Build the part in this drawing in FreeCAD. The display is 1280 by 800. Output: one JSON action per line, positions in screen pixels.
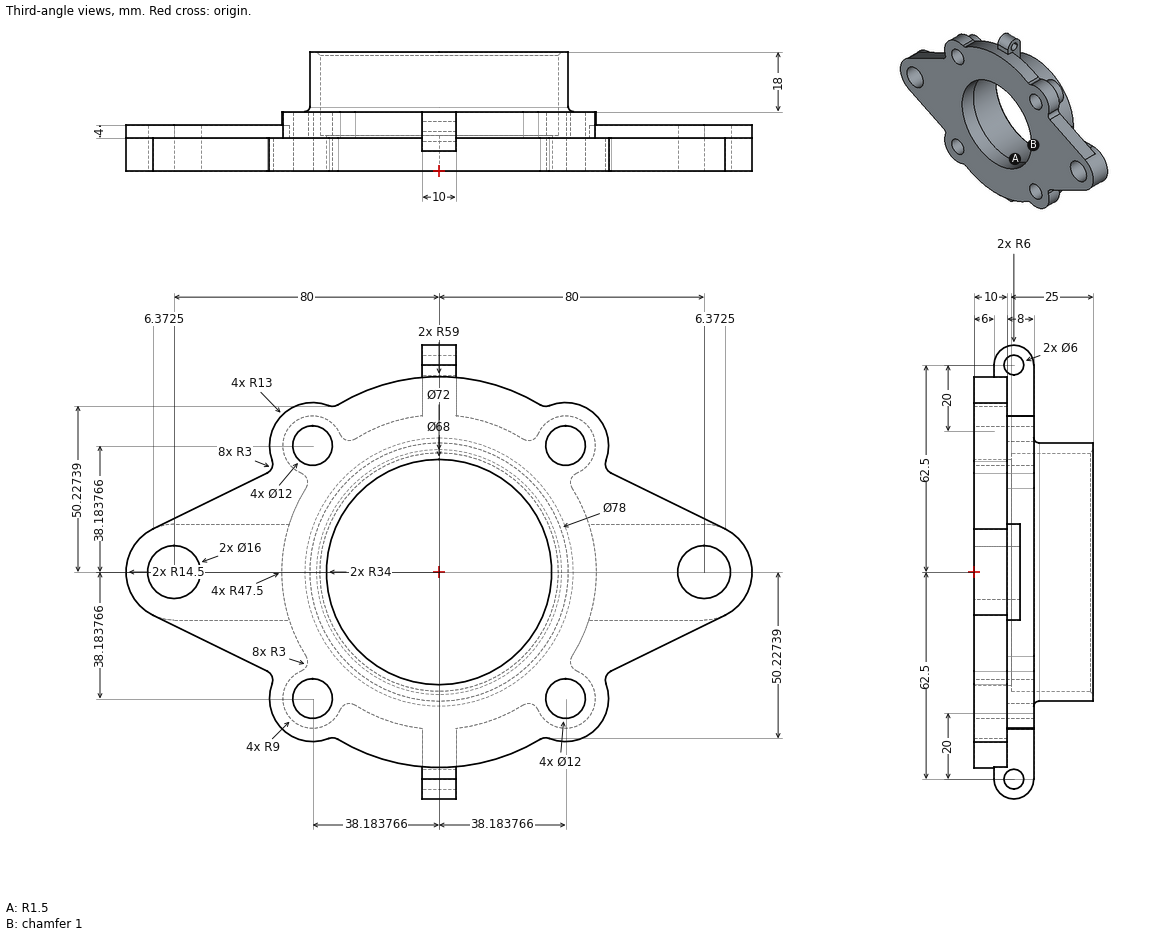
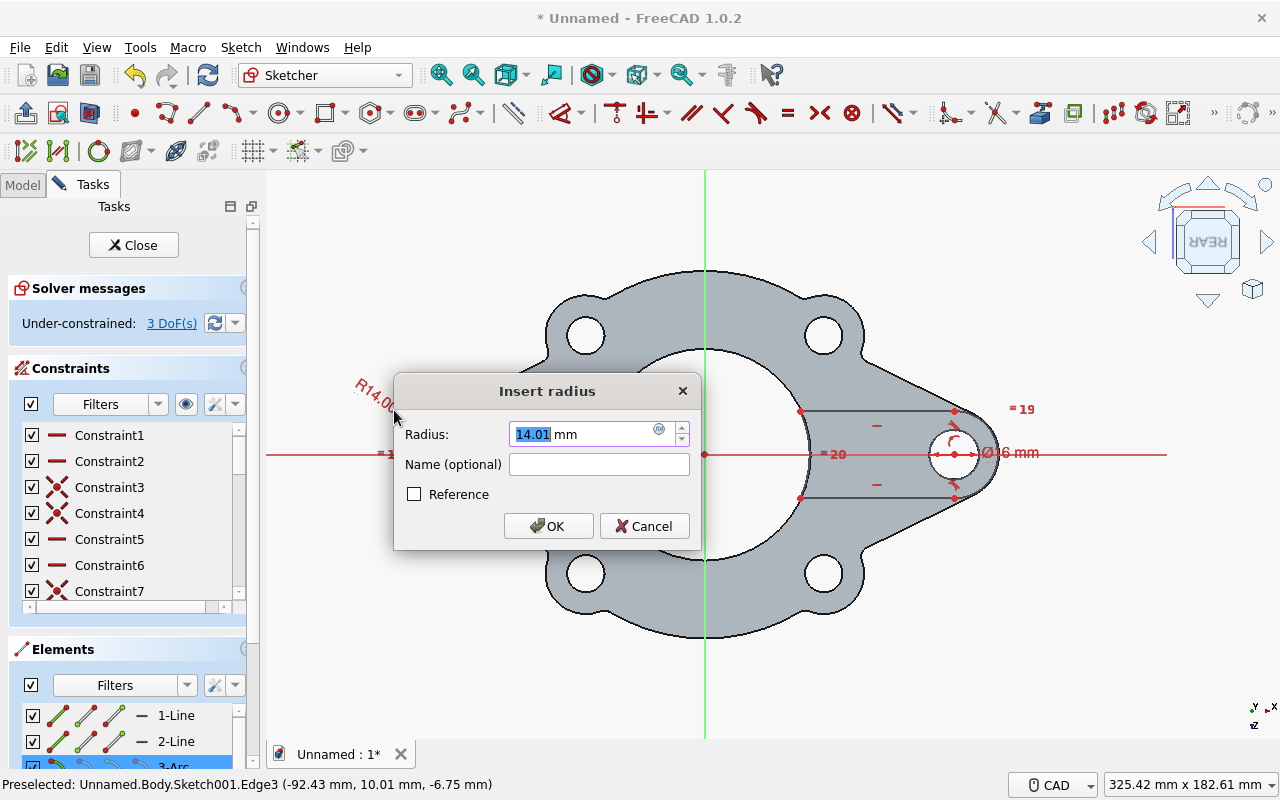
{"action": "type", "text": "14.5"}
{"action": "key", "text": "Return"}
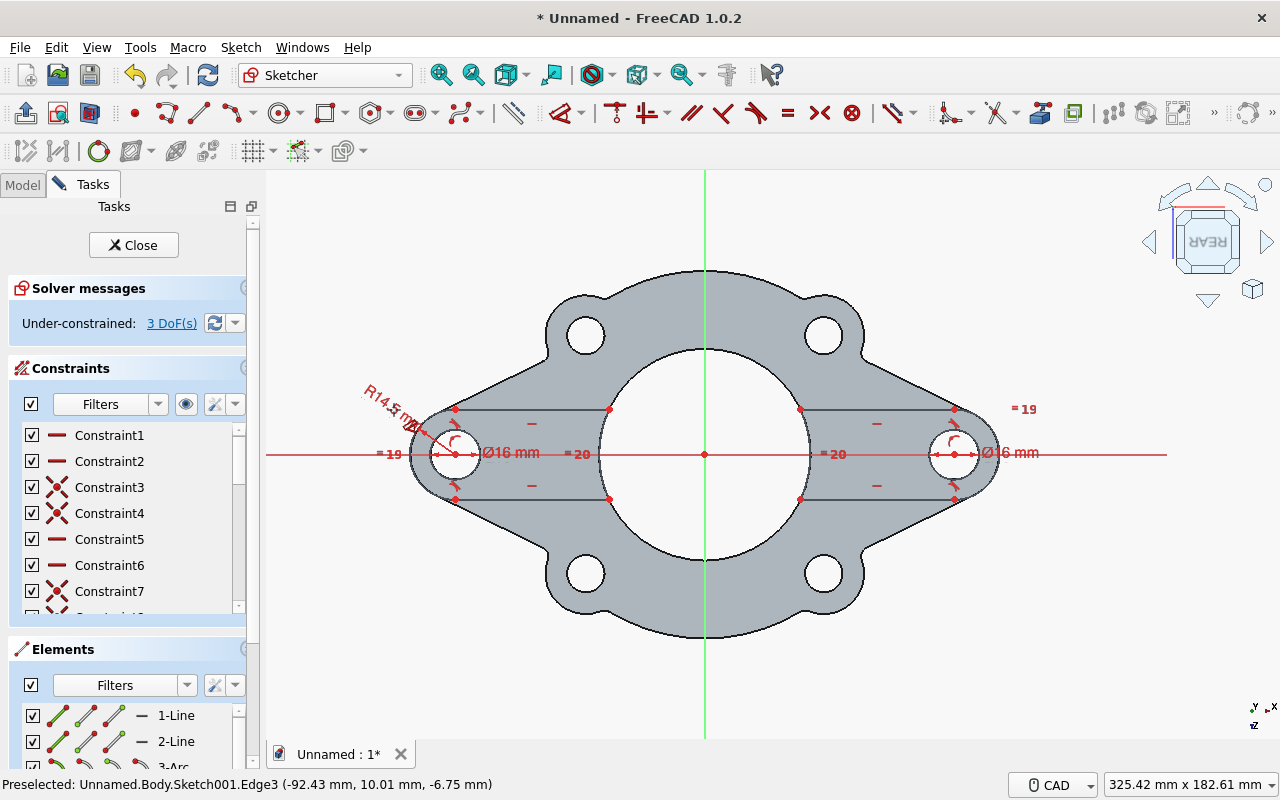
{"action": "left_click", "coordinate": [601, 436]}
{"action": "left_click", "coordinate": [570, 430]}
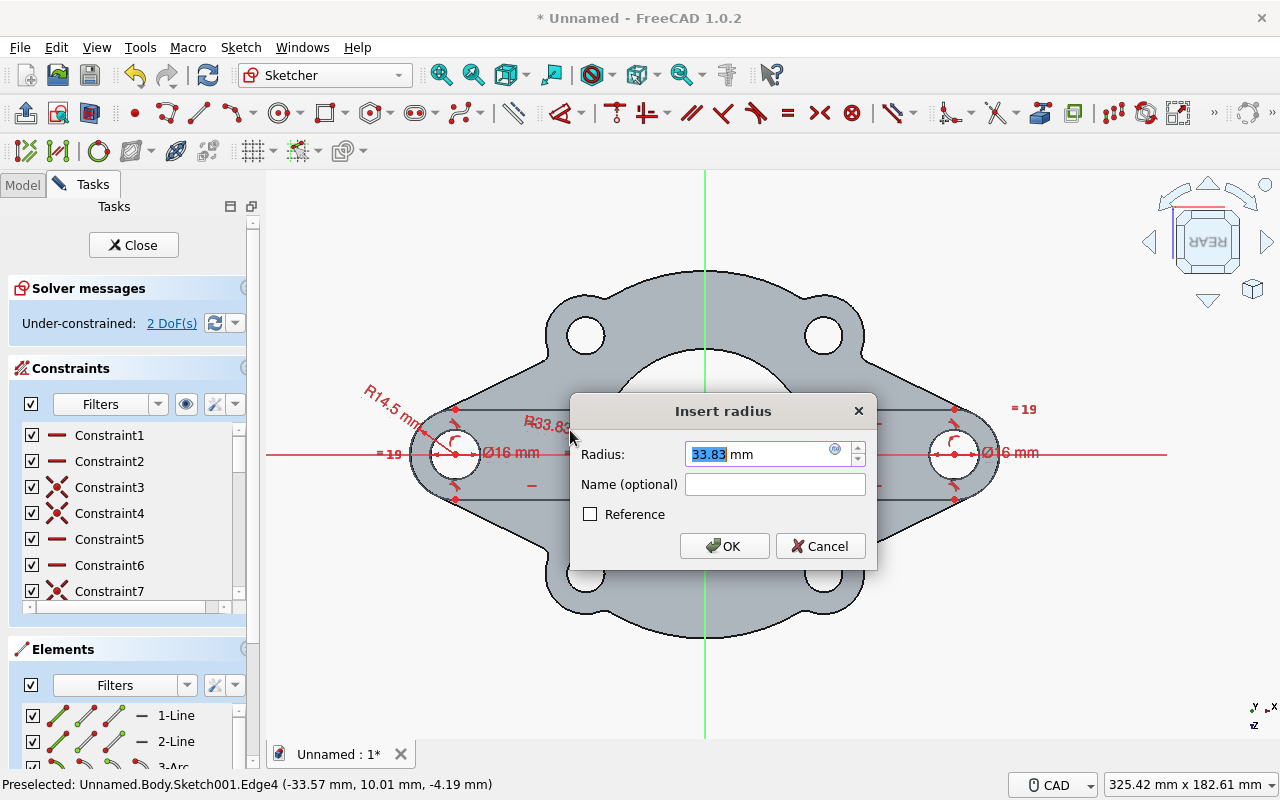
{"action": "type", "text": "34"}
{"action": "key", "text": "Return"}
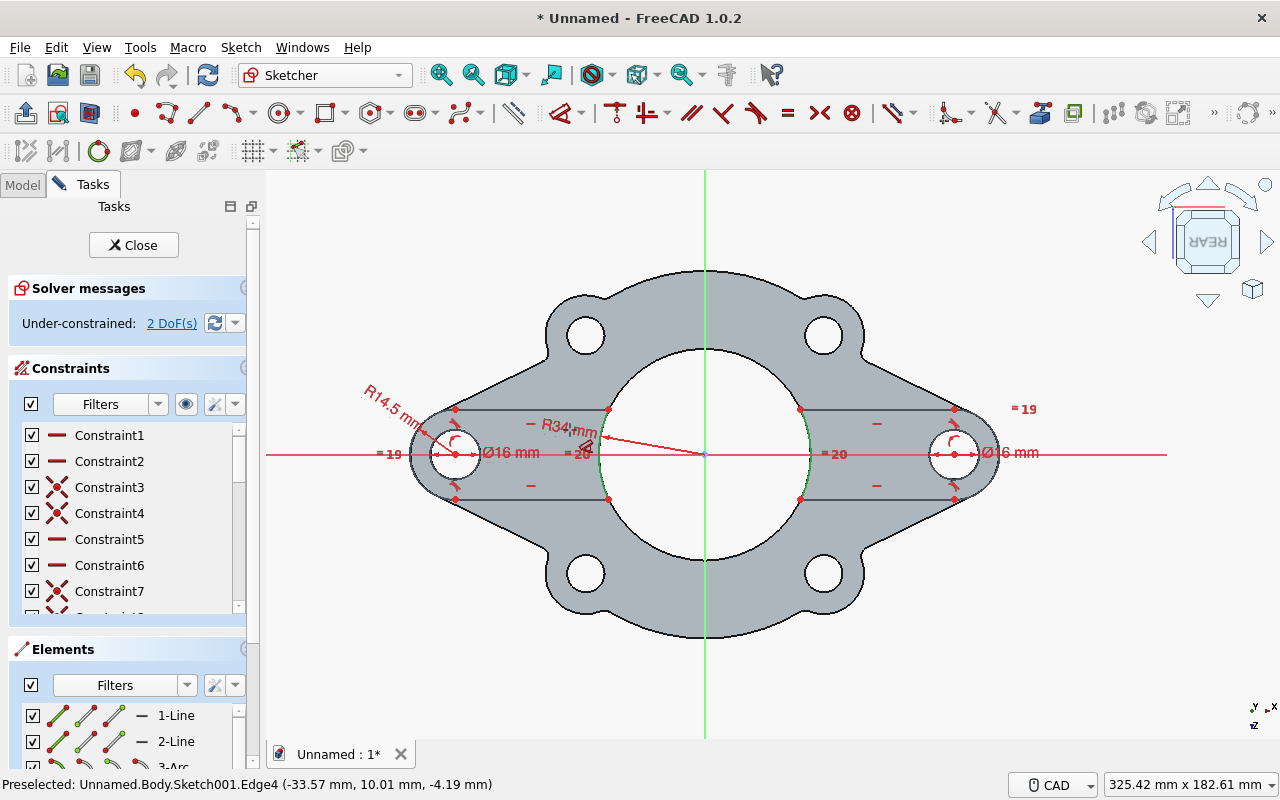
{"action": "left_click", "coordinate": [455, 455]}
{"action": "left_click", "coordinate": [637, 489]}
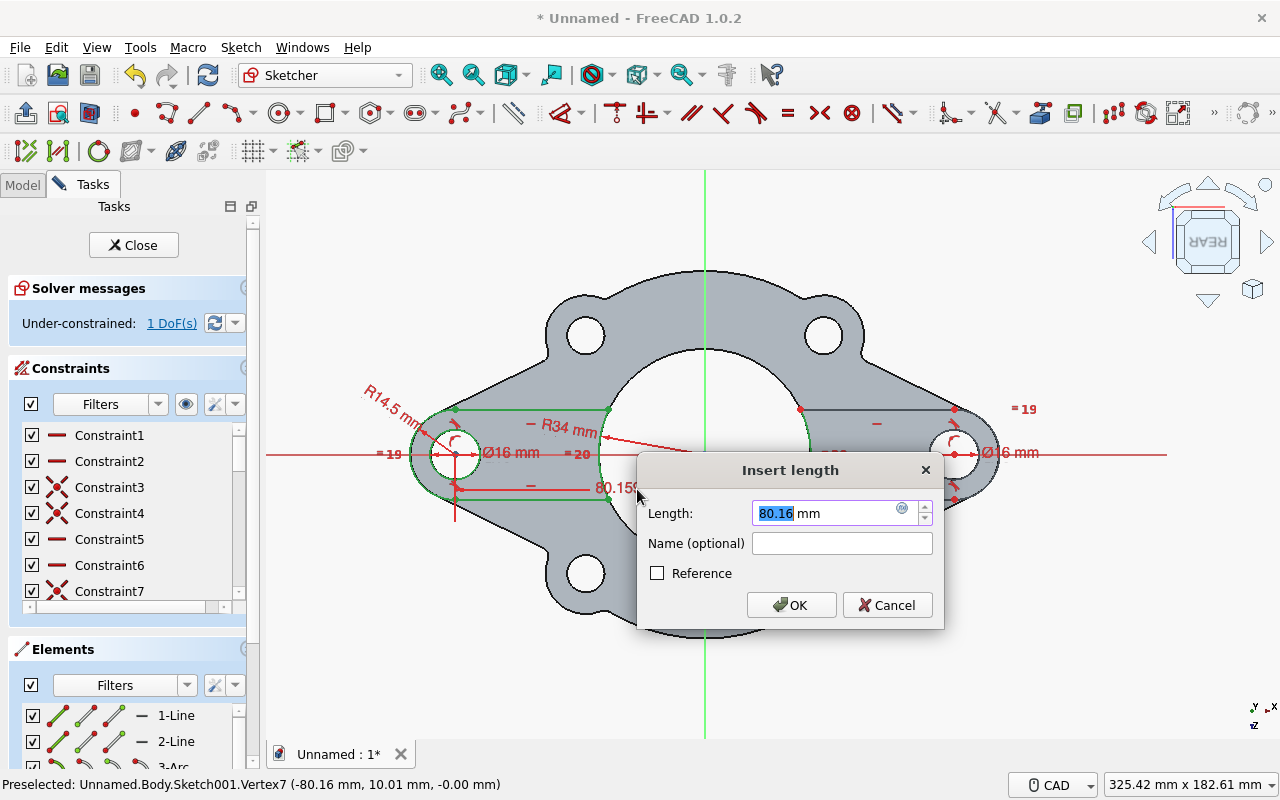
{"action": "type", "text": "80"}
{"action": "key", "text": "Return"}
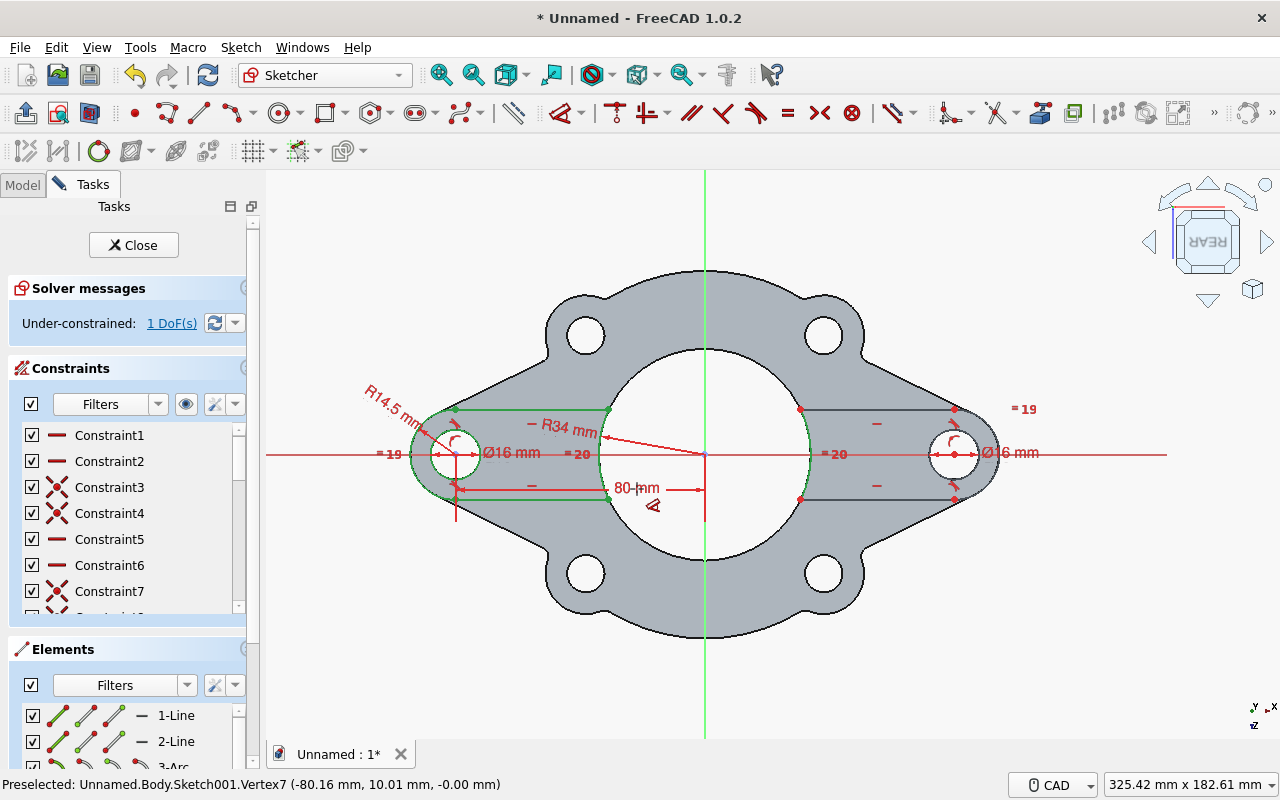
{"action": "left_click", "coordinate": [954, 455]}
{"action": "left_click", "coordinate": [772, 489]}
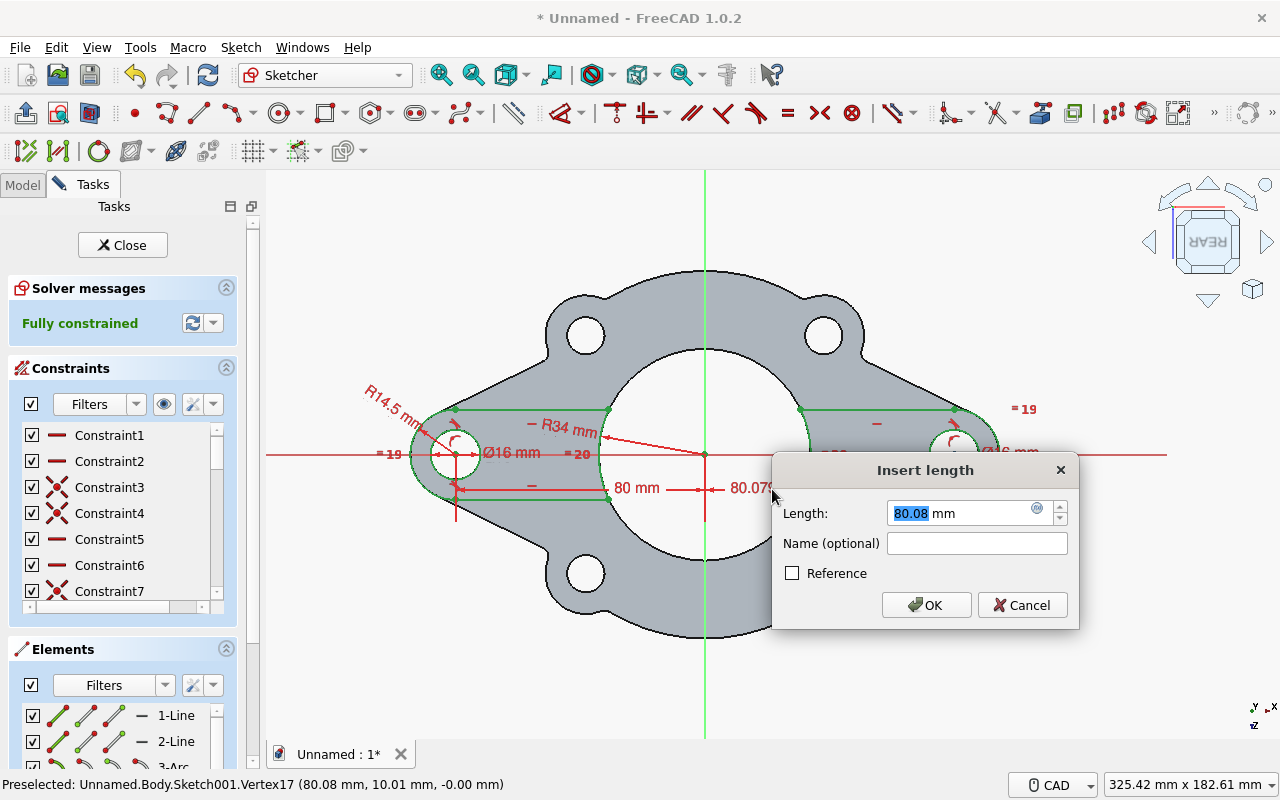
{"action": "type", "text": "80"}
{"action": "key", "text": "Return"}
{"action": "key", "text": "Escape"}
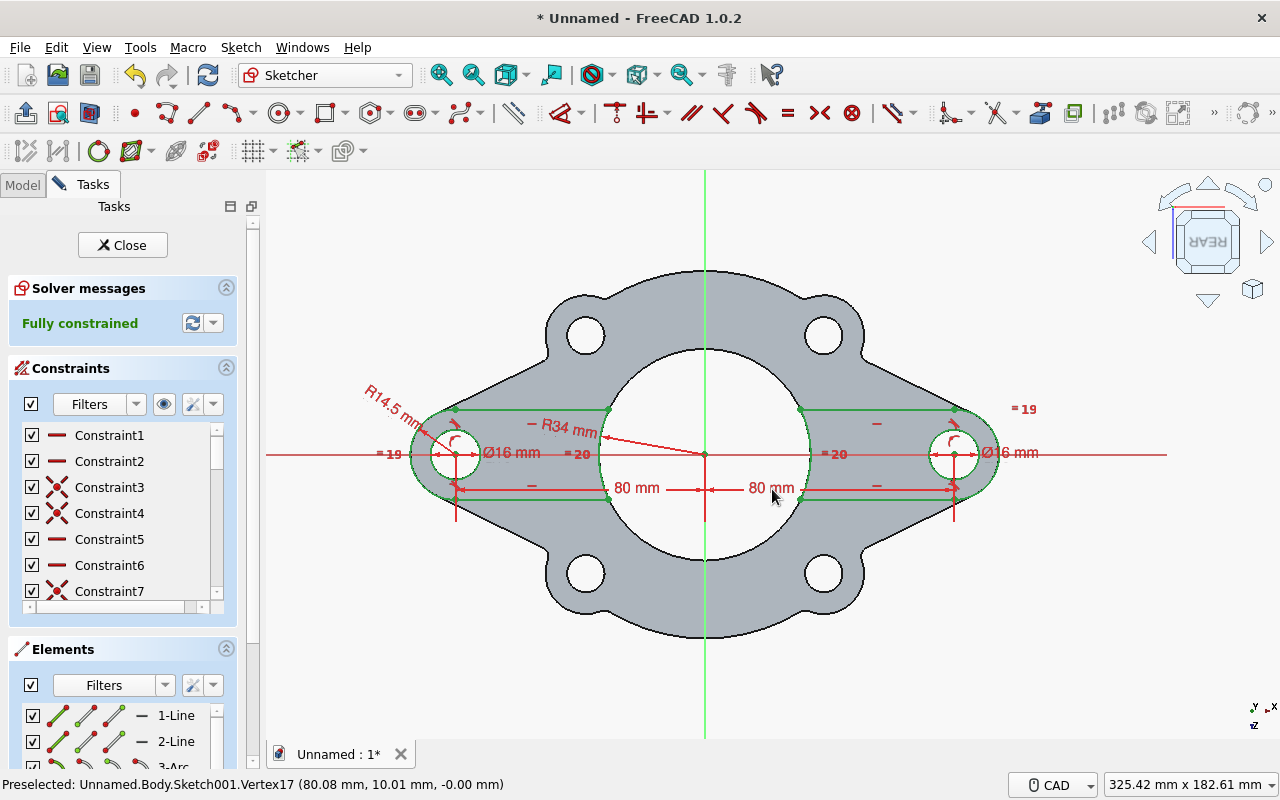
{"action": "left_click", "coordinate": [123, 245]}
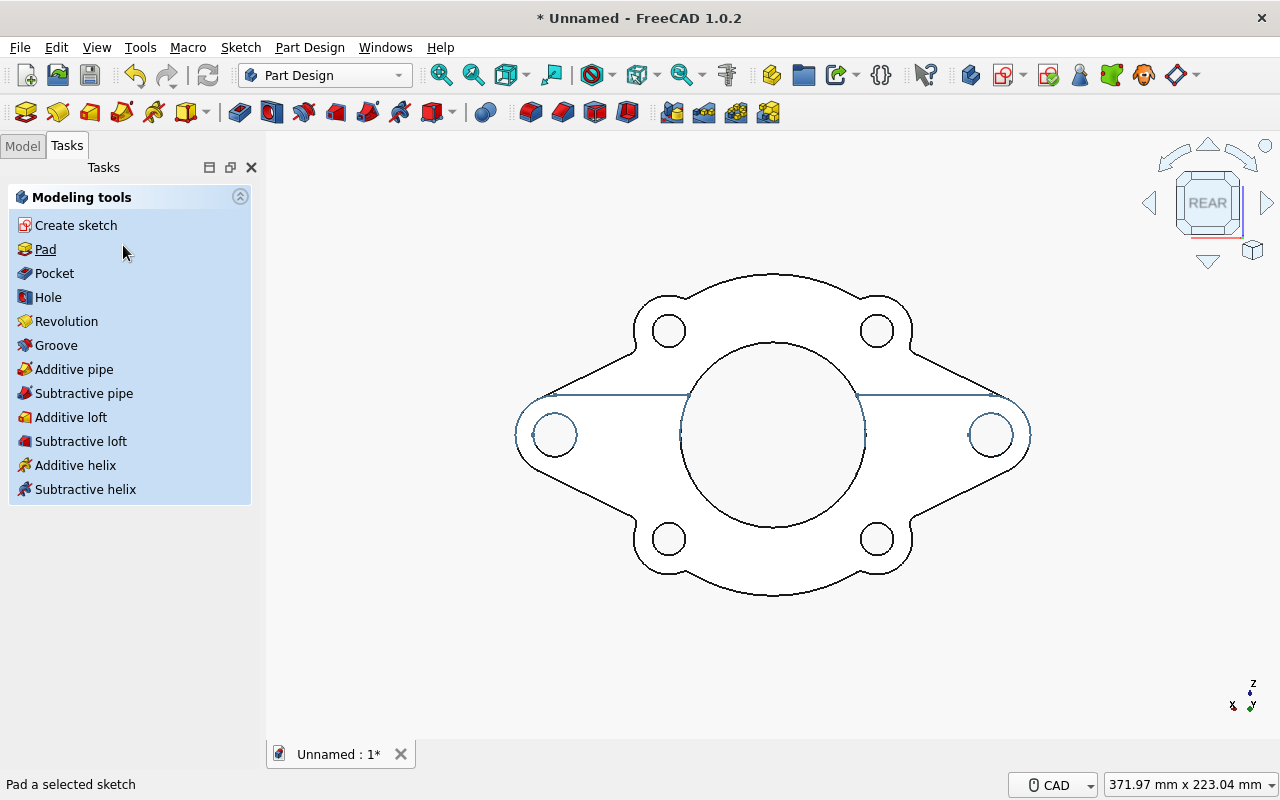
{"action": "left_click", "coordinate": [26, 112]}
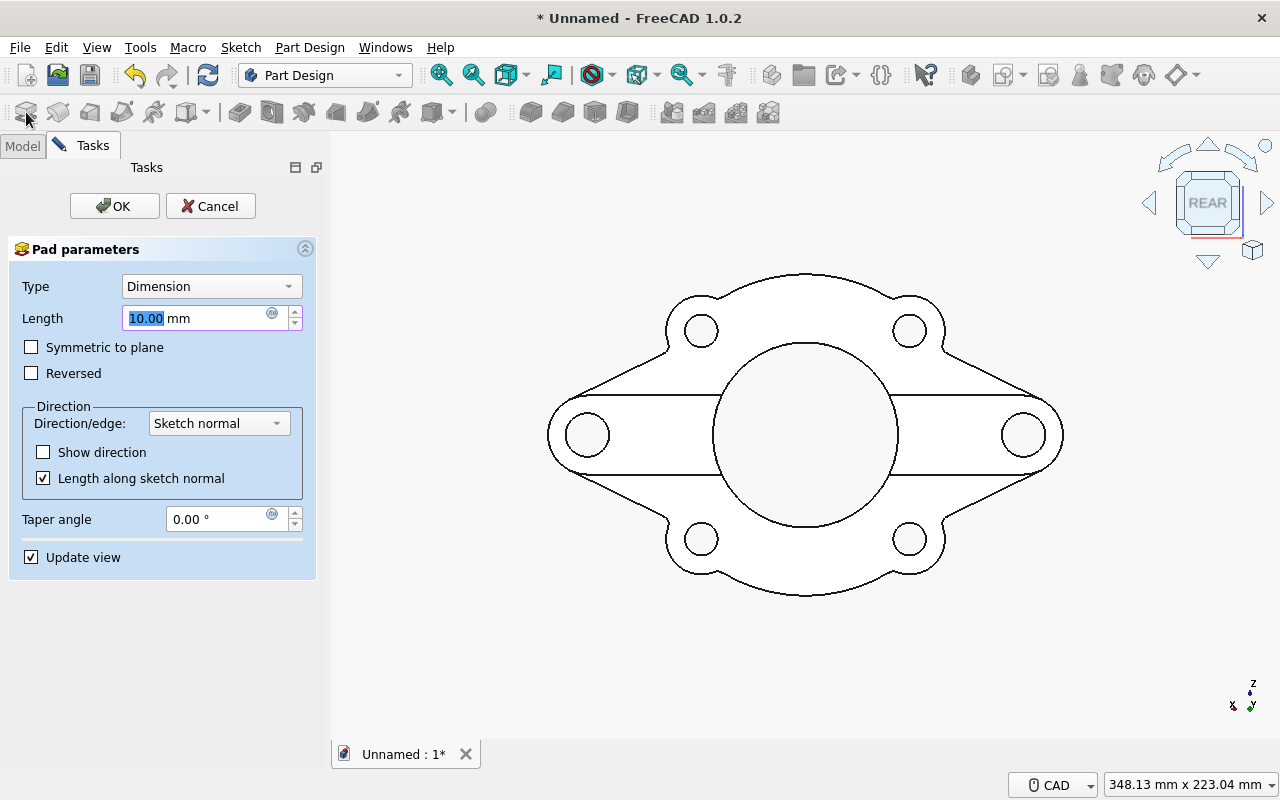
{"action": "type", "text": "4"}
{"action": "key", "text": "Tab"}